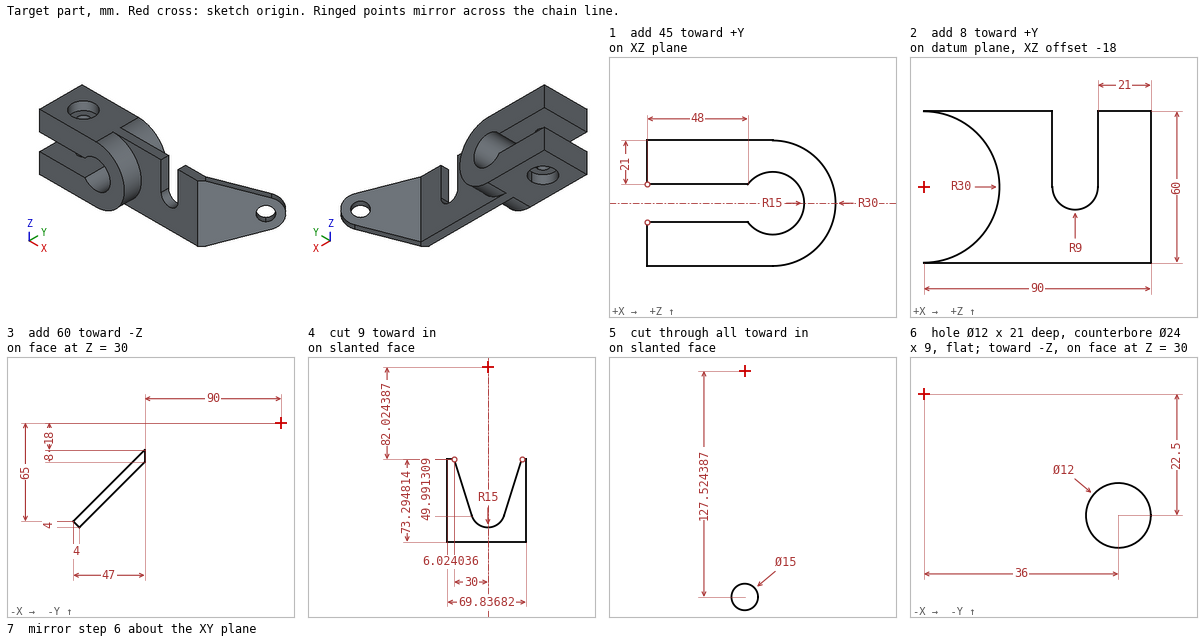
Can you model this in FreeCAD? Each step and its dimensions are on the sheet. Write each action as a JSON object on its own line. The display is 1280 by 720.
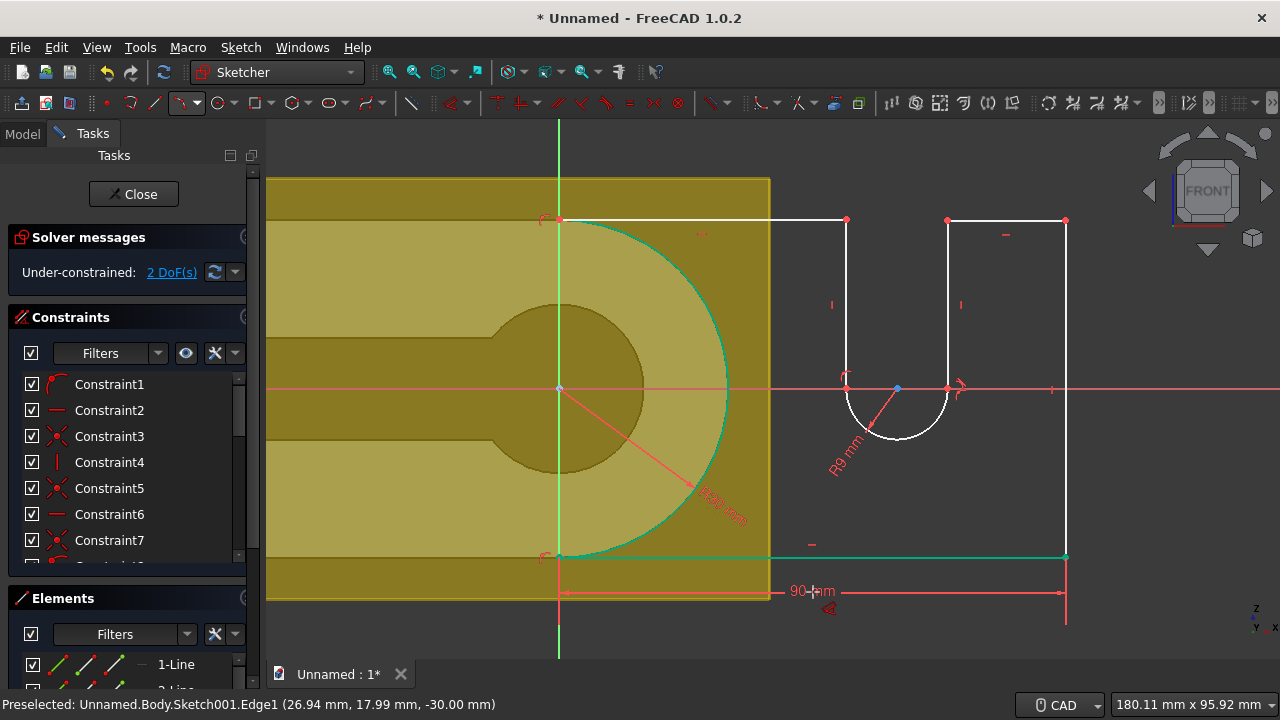
{"action": "left_click", "coordinate": [1066, 457]}
{"action": "left_click", "coordinate": [1100, 312]}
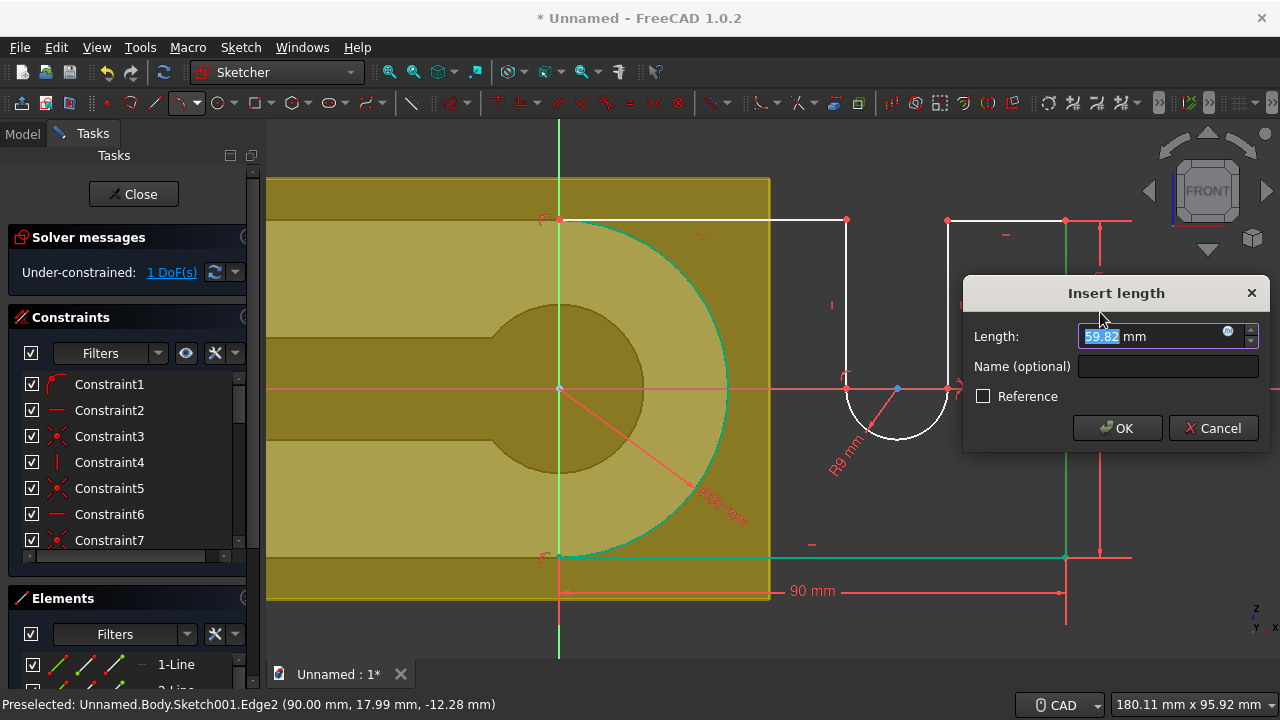
{"action": "type", "text": "60"}
{"action": "key", "text": "Return"}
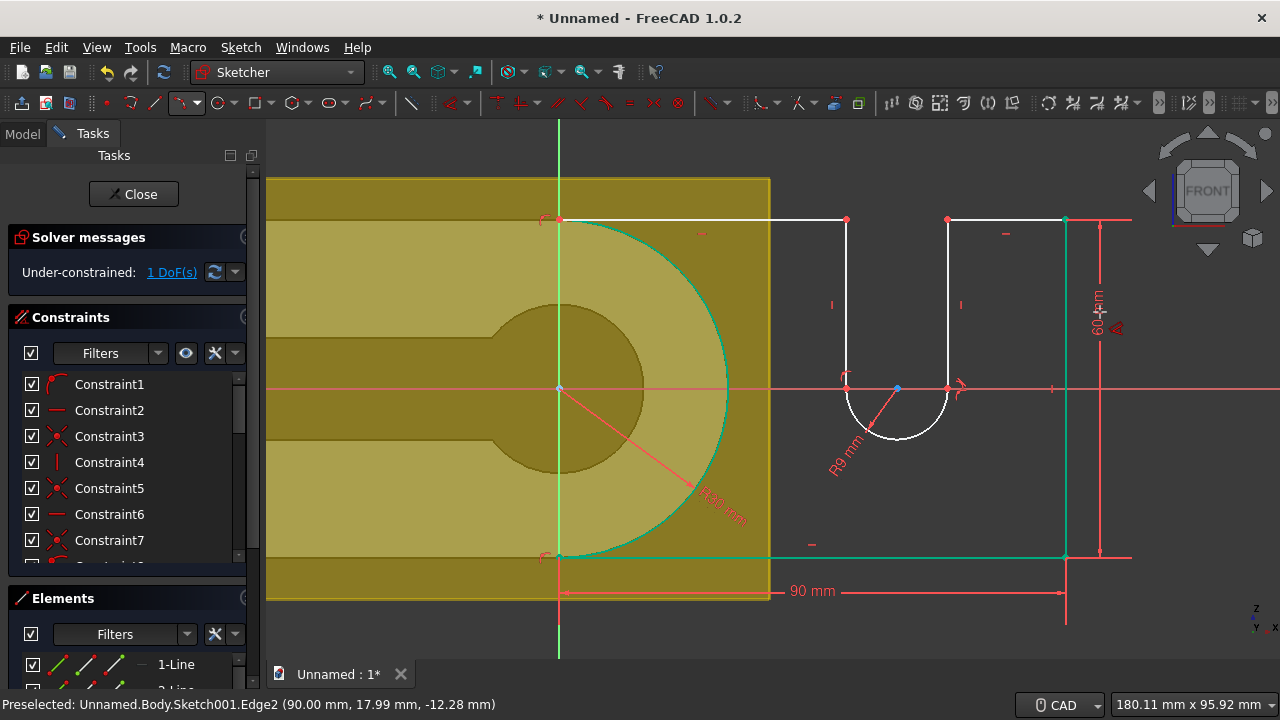
{"action": "left_click", "coordinate": [1030, 220]}
{"action": "left_click", "coordinate": [1007, 186]}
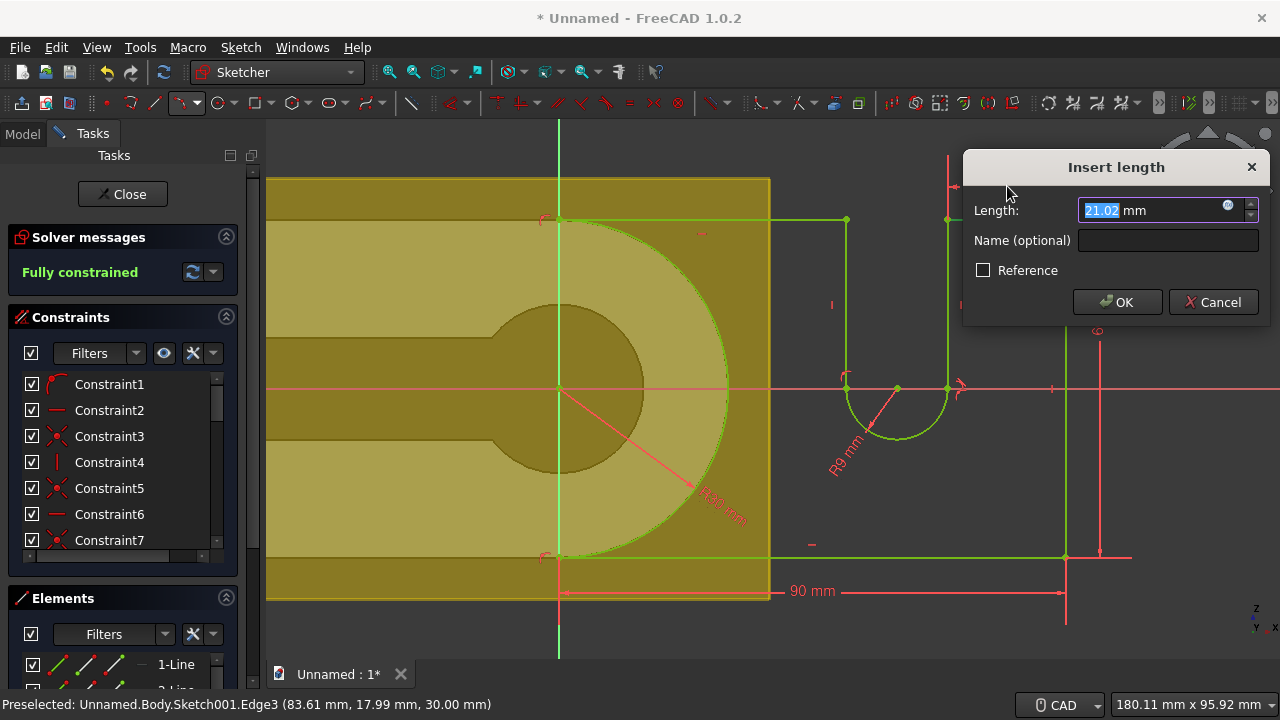
{"action": "type", "text": "21"}
{"action": "key", "text": "Return"}
{"action": "key", "text": "Escape"}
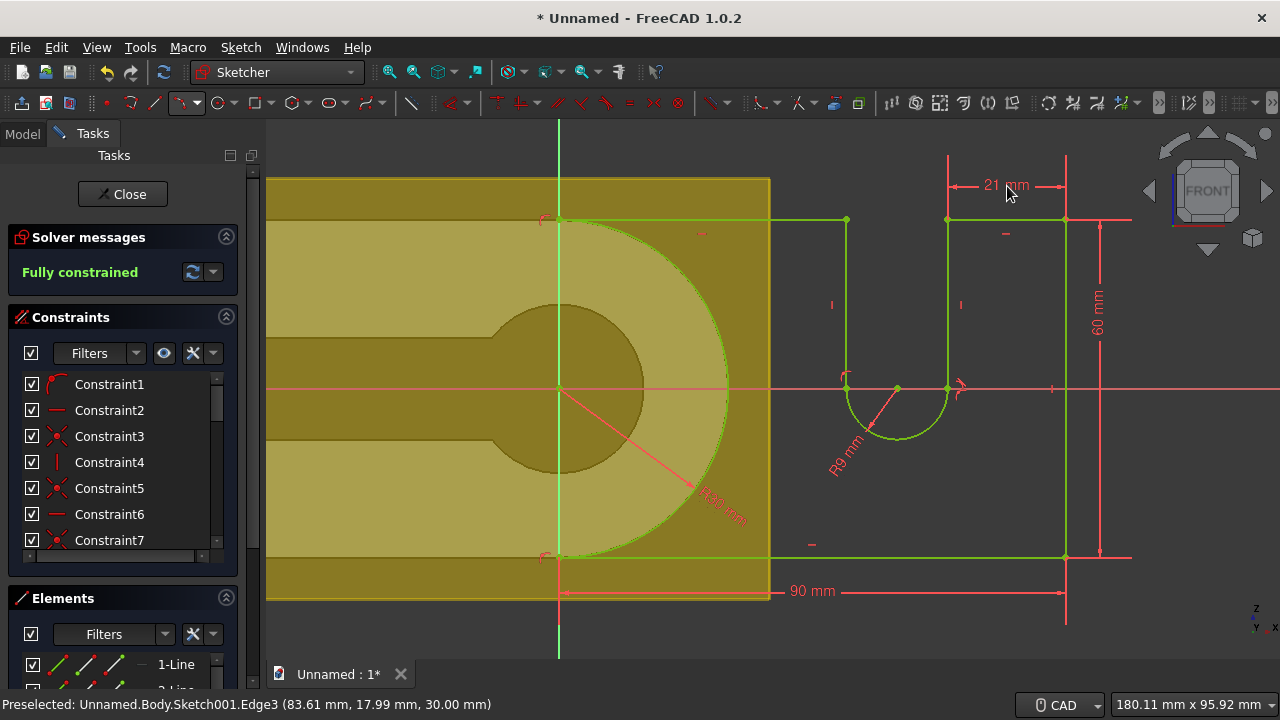
{"action": "left_click", "coordinate": [123, 194]}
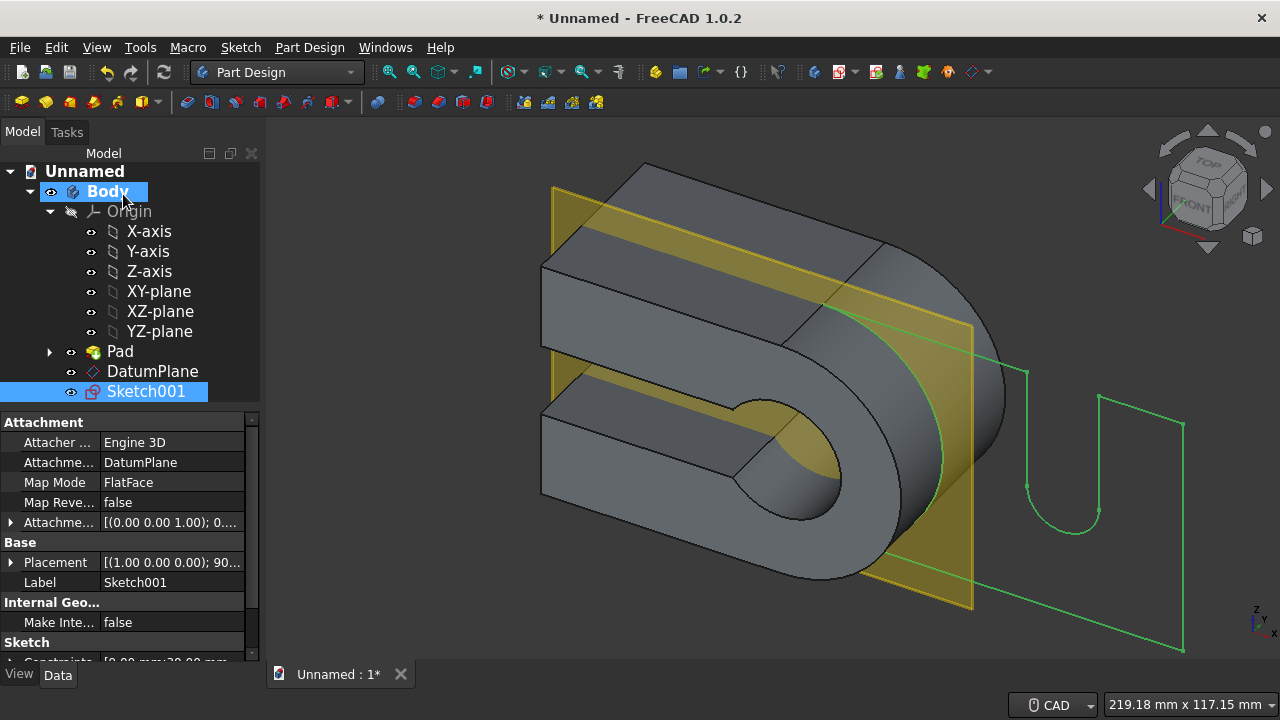
{"action": "left_click", "coordinate": [22, 102]}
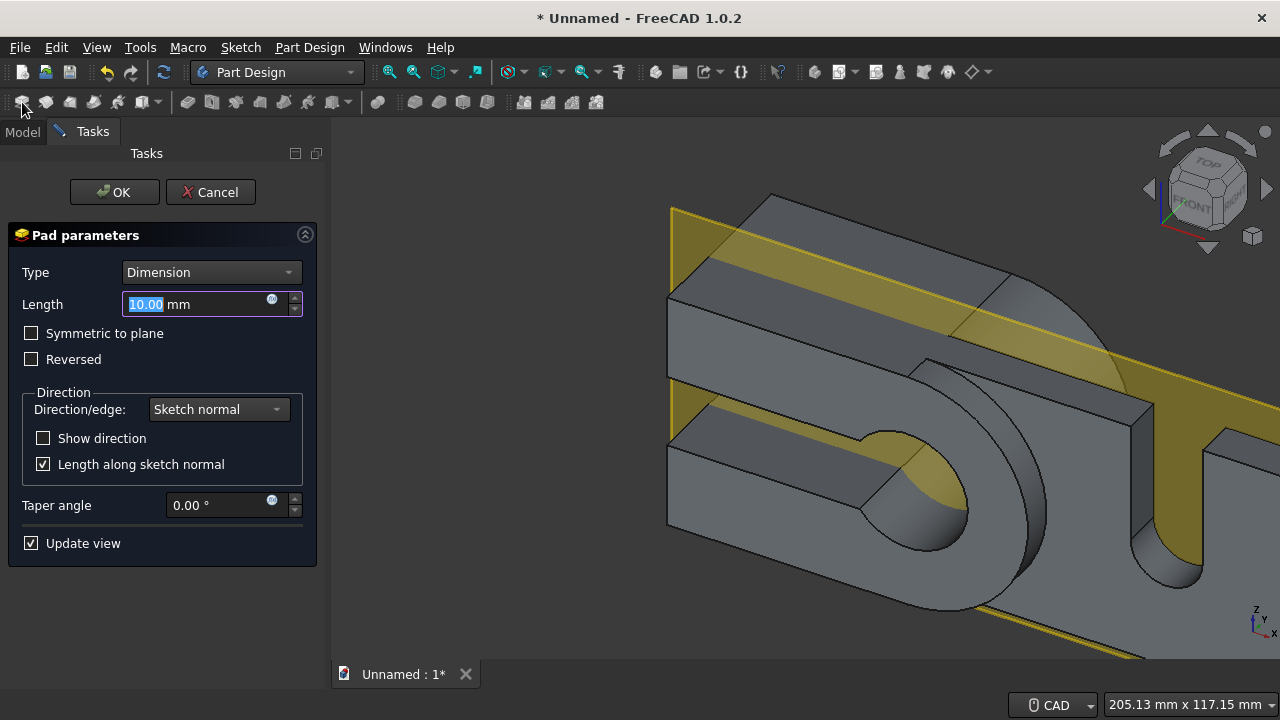
{"action": "type", "text": "8"}
{"action": "key", "text": "Tab"}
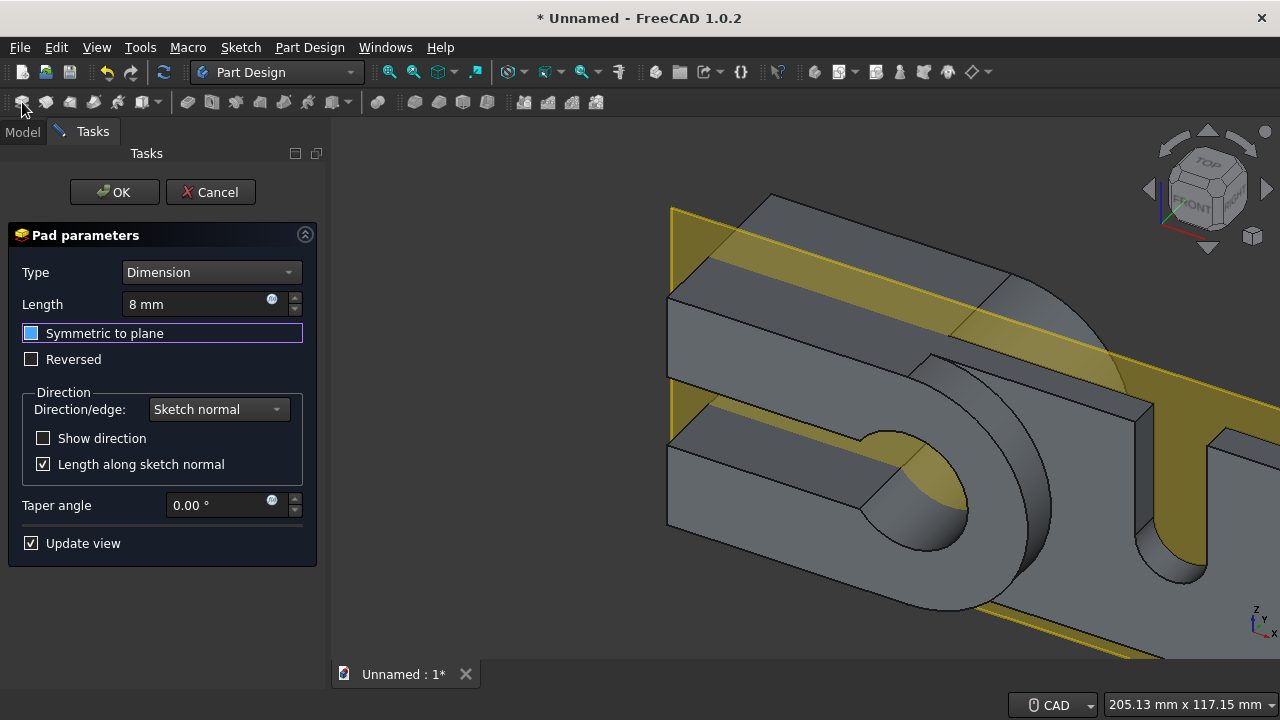
{"action": "left_click", "coordinate": [30, 359]}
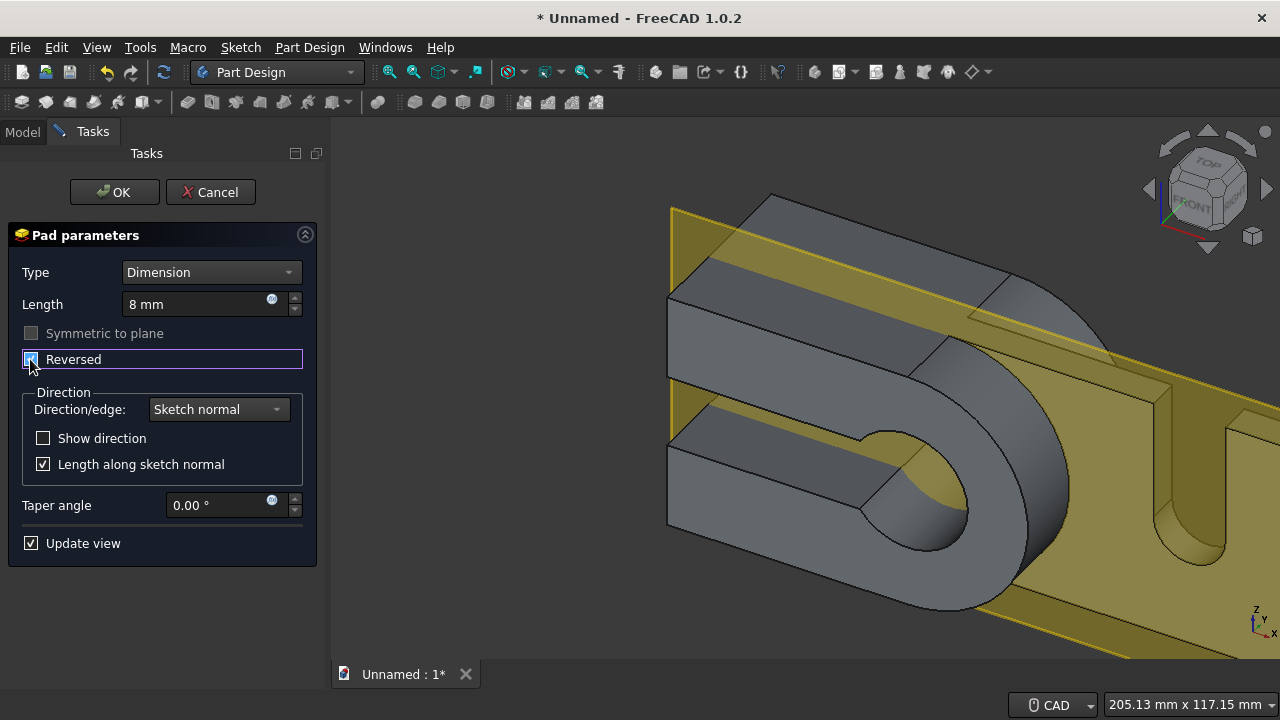
{"action": "left_click", "coordinate": [115, 192]}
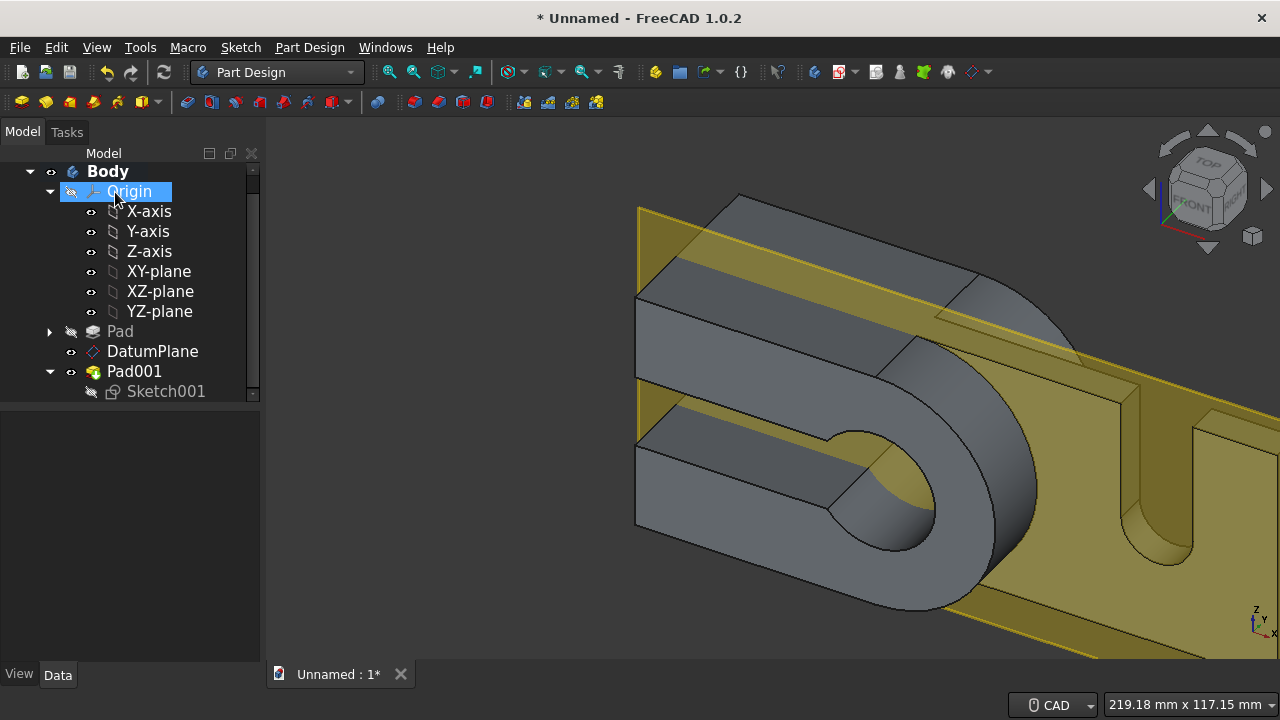
{"action": "left_click", "coordinate": [116, 352]}
{"action": "key", "text": "space"}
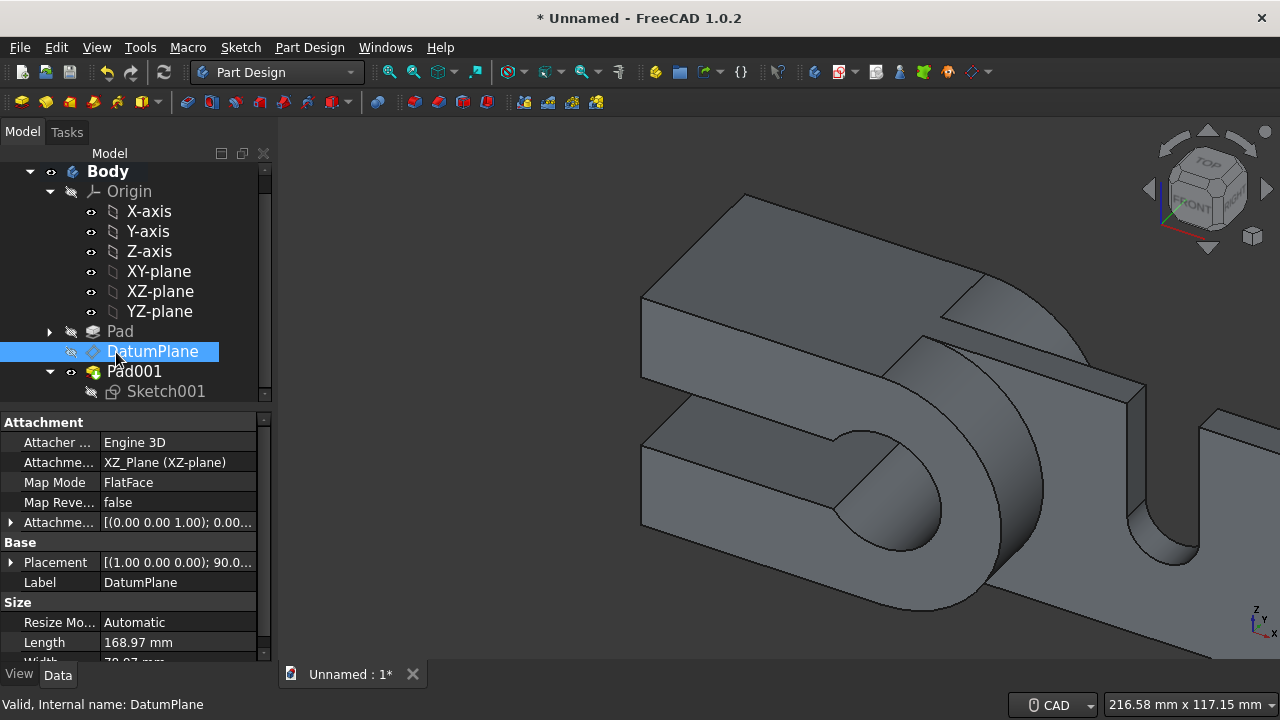
{"action": "key", "text": "v f"}